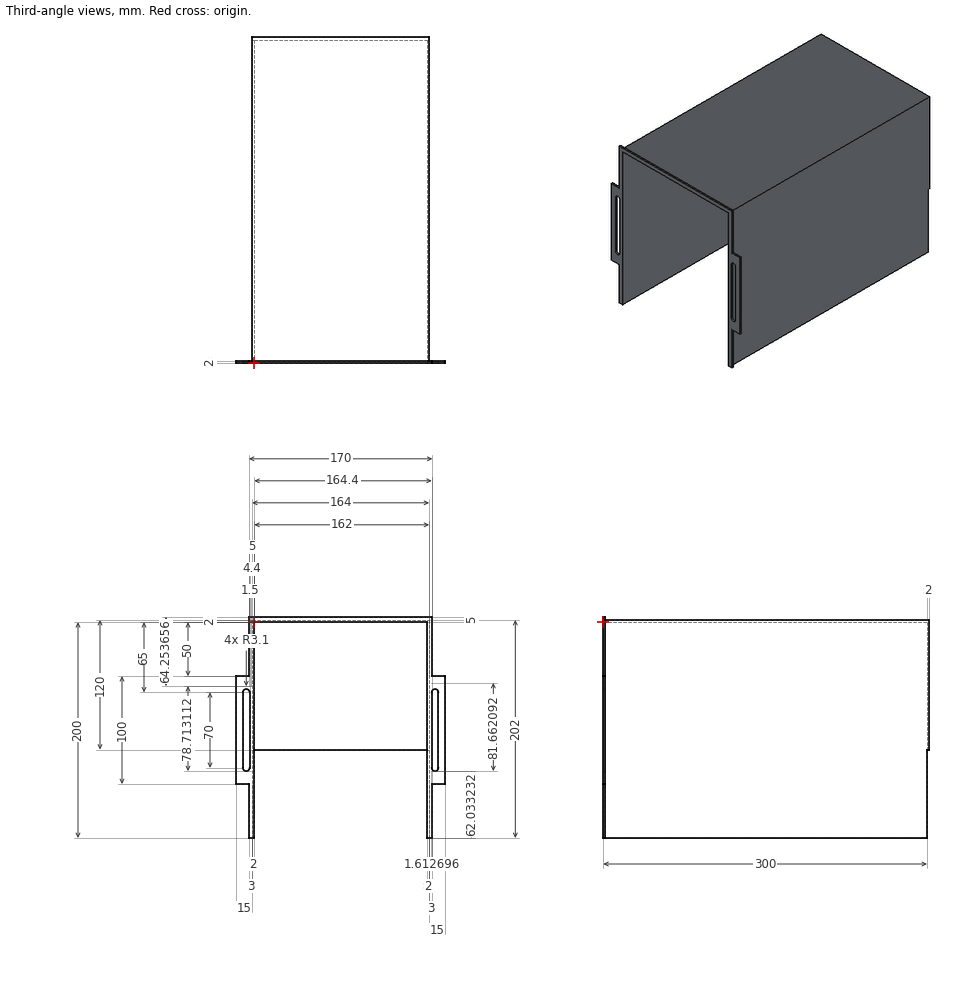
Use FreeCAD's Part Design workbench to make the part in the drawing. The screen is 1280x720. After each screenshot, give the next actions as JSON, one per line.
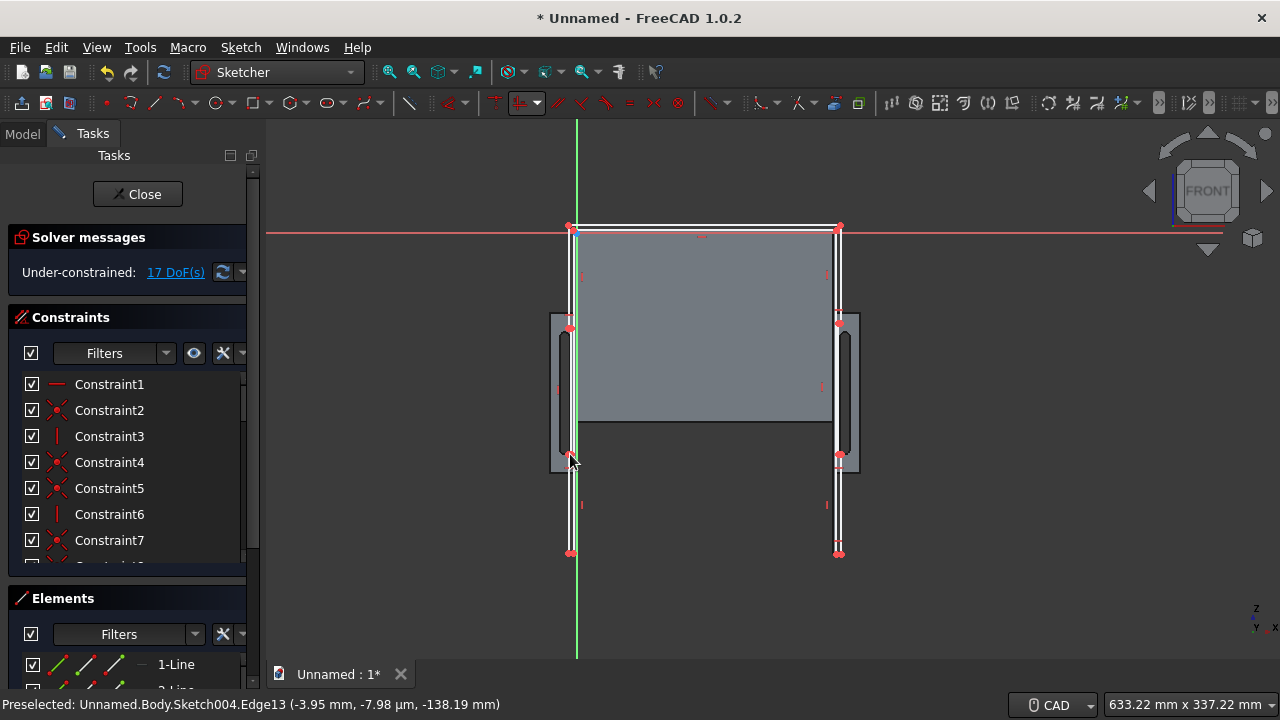
{"action": "scroll", "coordinate": [570, 554], "scroll_direction": "up", "scroll_amount": 12}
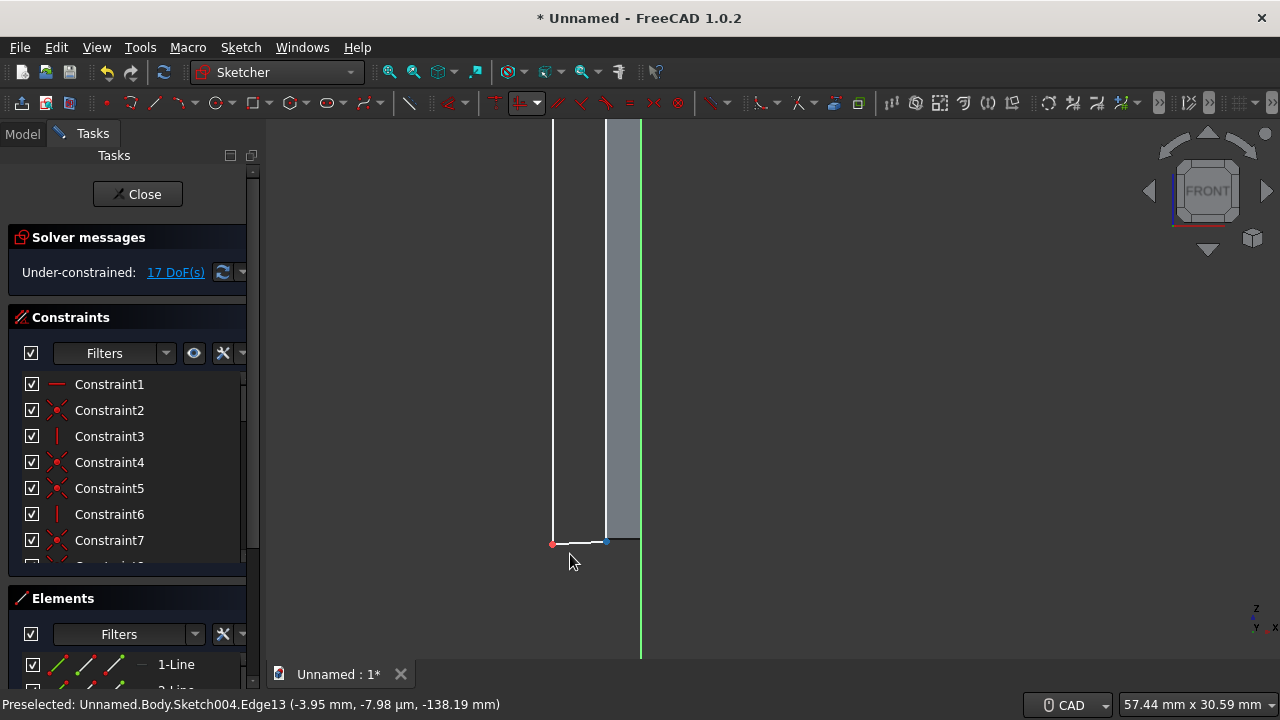
{"action": "left_click", "coordinate": [569, 544]}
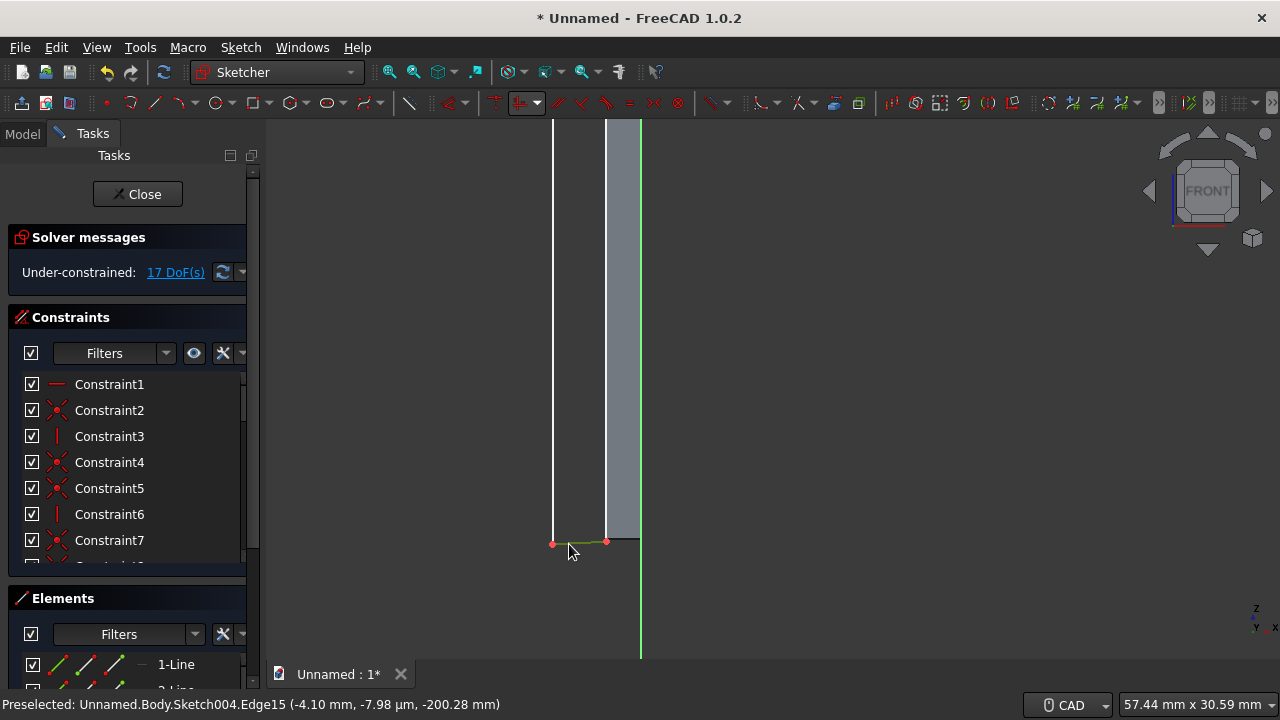
{"action": "left_click", "coordinate": [540, 104]}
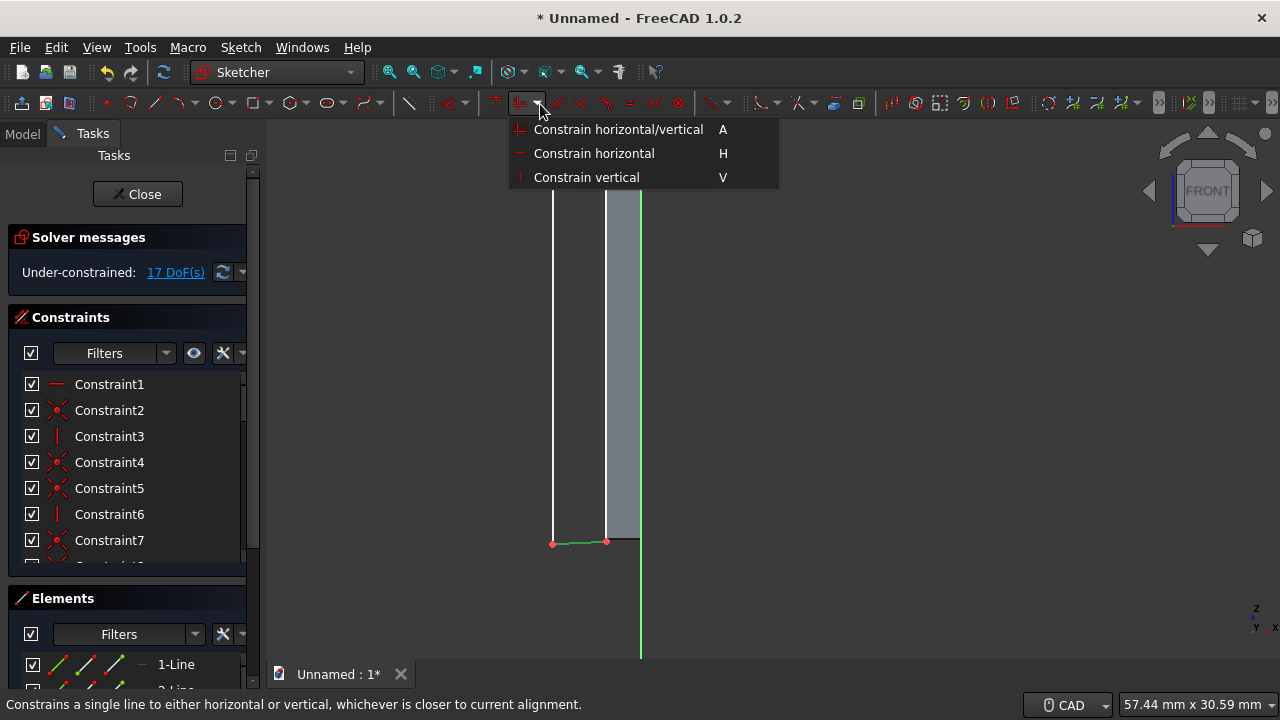
{"action": "left_click", "coordinate": [644, 153]}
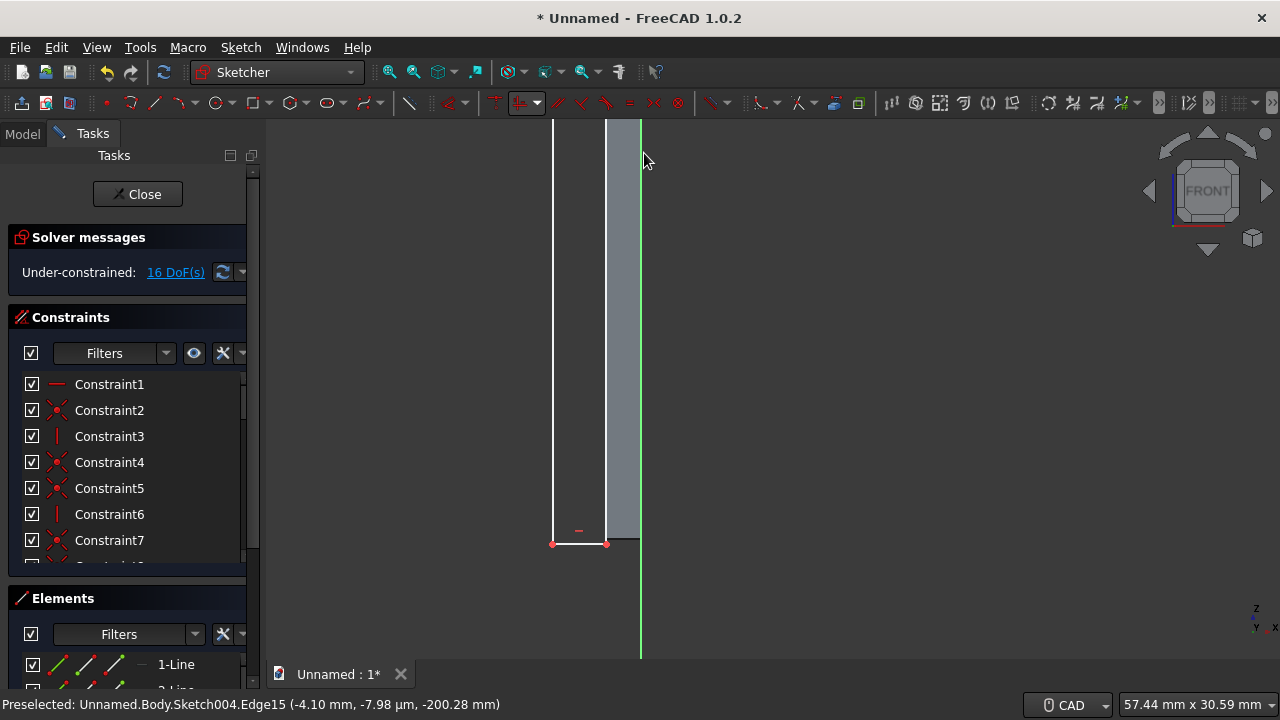
{"action": "left_click", "coordinate": [448, 104]}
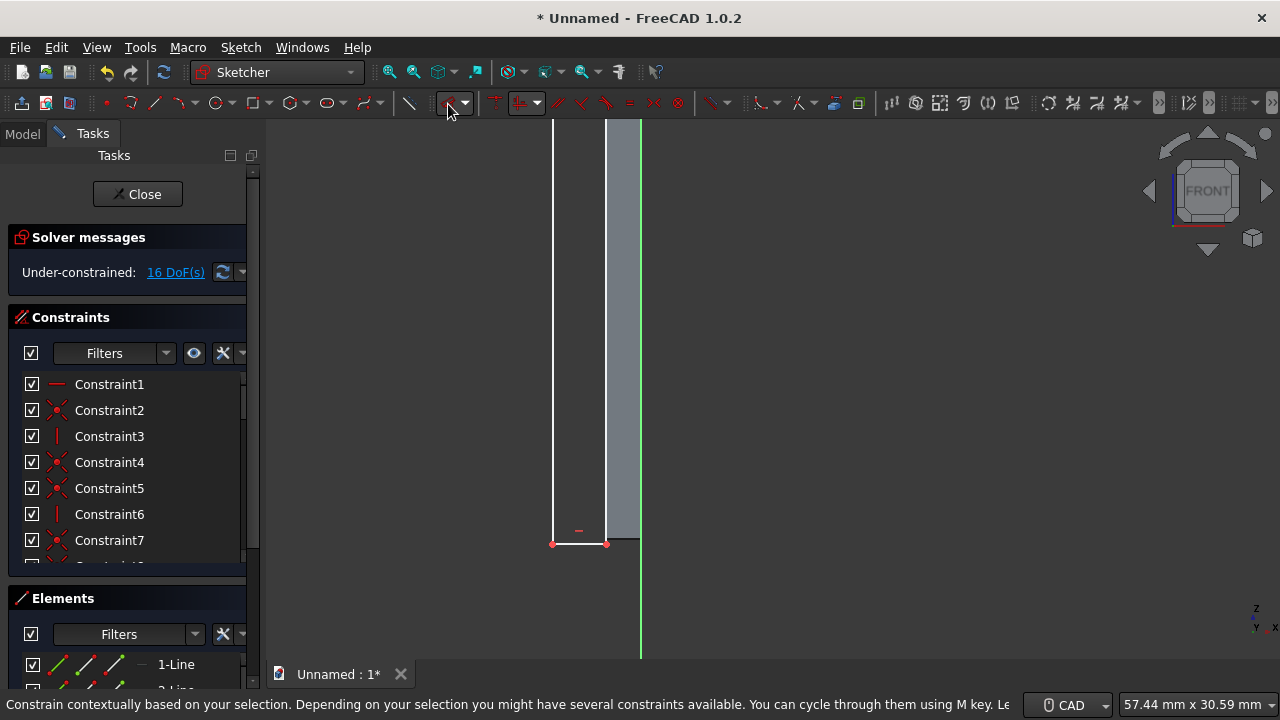
{"action": "scroll", "coordinate": [570, 555], "scroll_direction": "down", "scroll_amount": 12}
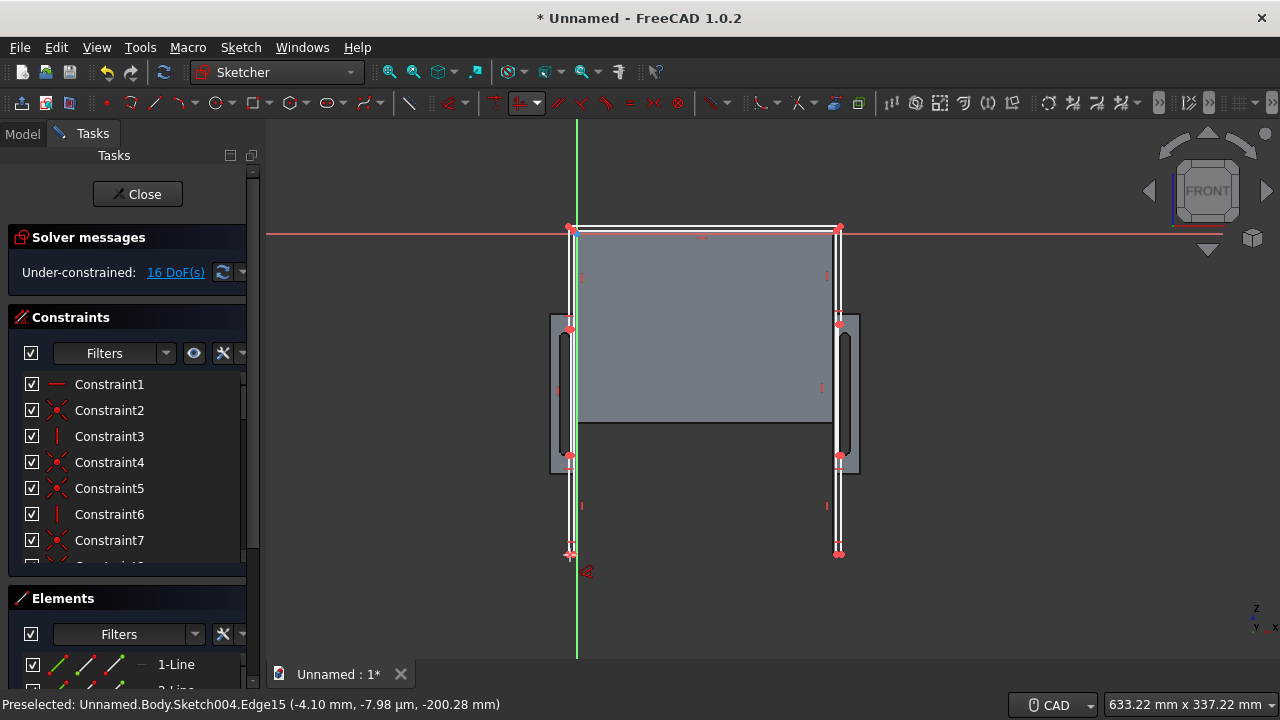
{"action": "scroll", "coordinate": [838, 555], "scroll_direction": "up", "scroll_amount": 12}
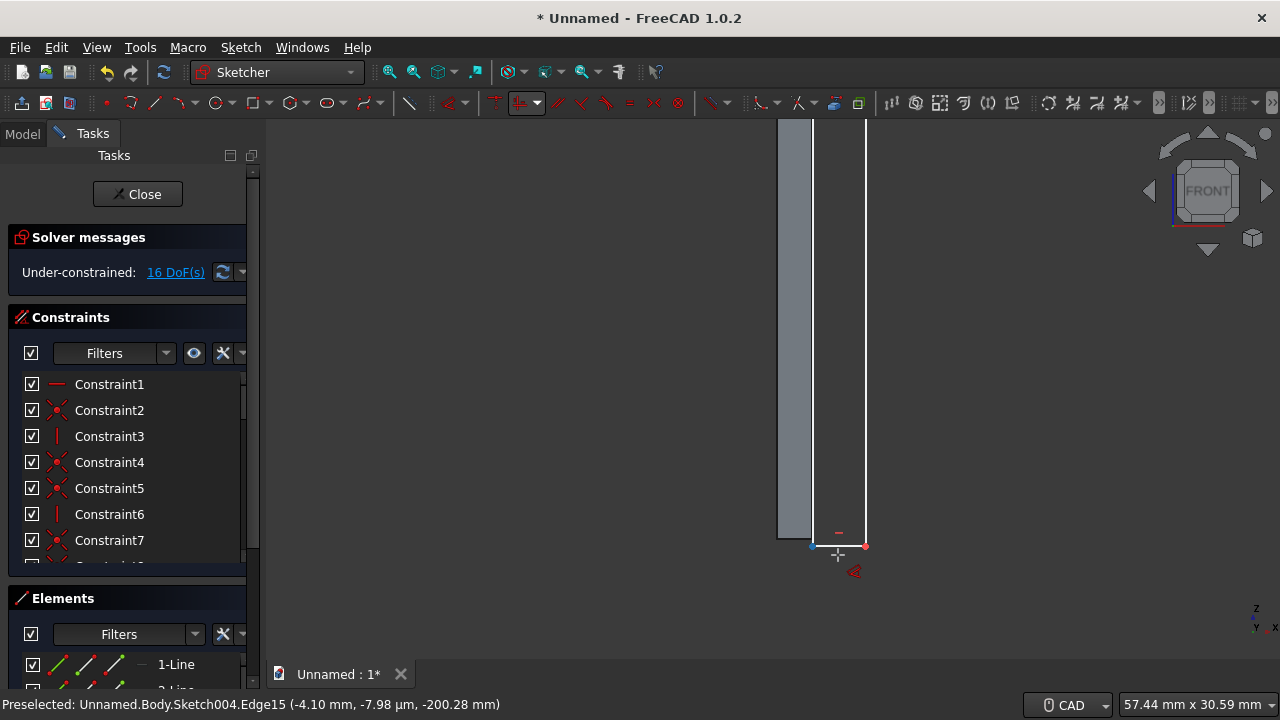
{"action": "left_click", "coordinate": [829, 546]}
{"action": "left_click", "coordinate": [839, 580]}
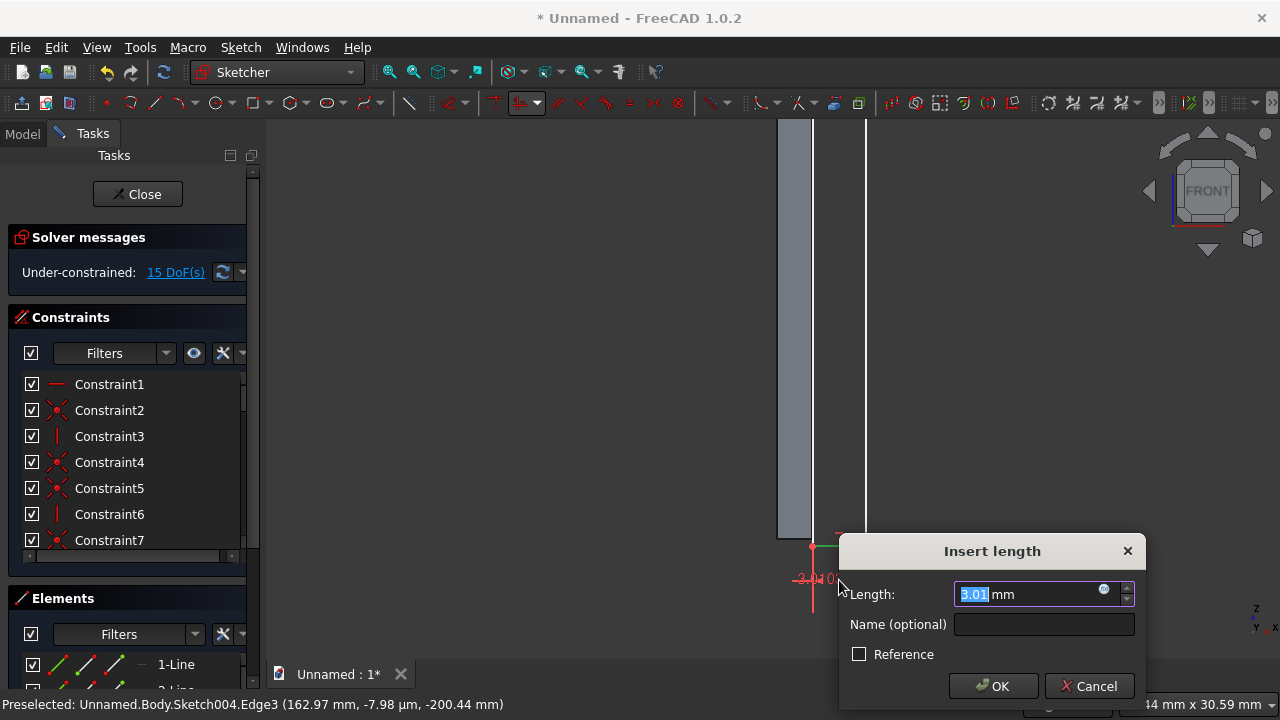
{"action": "type", "text": "3"}
{"action": "key", "text": "Return"}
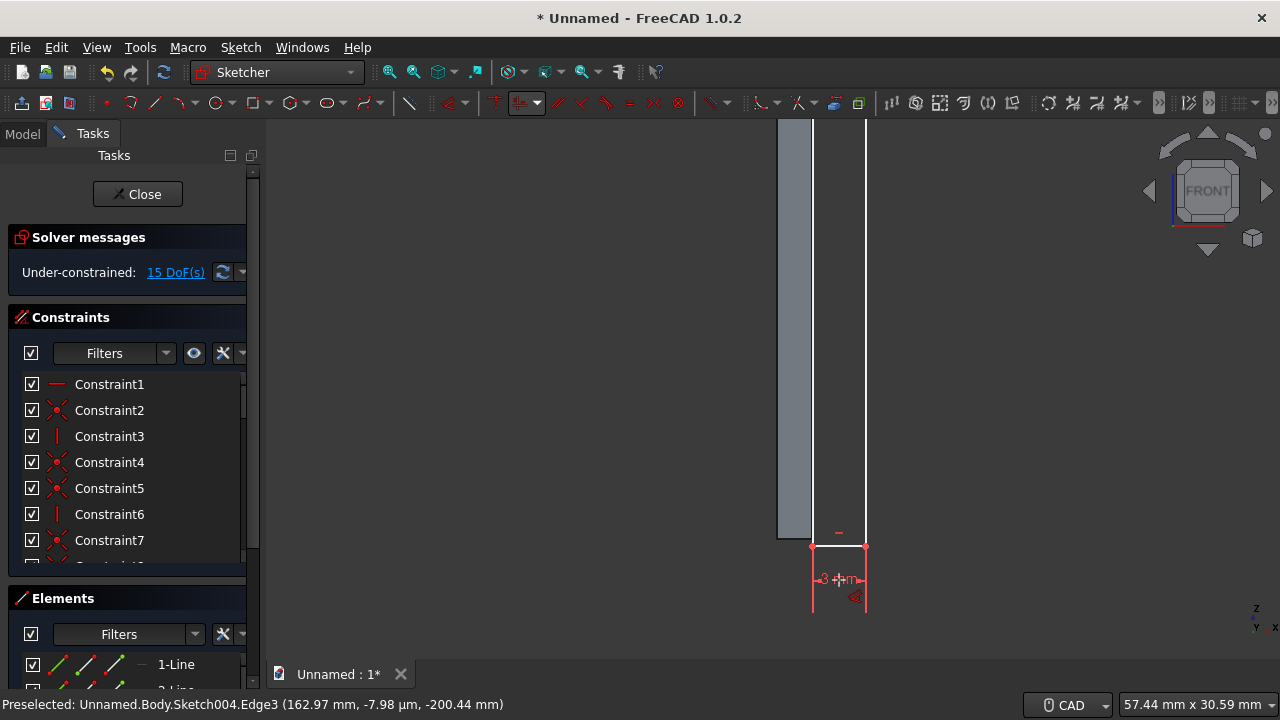
{"action": "scroll", "coordinate": [838, 555], "scroll_direction": "down", "scroll_amount": 12}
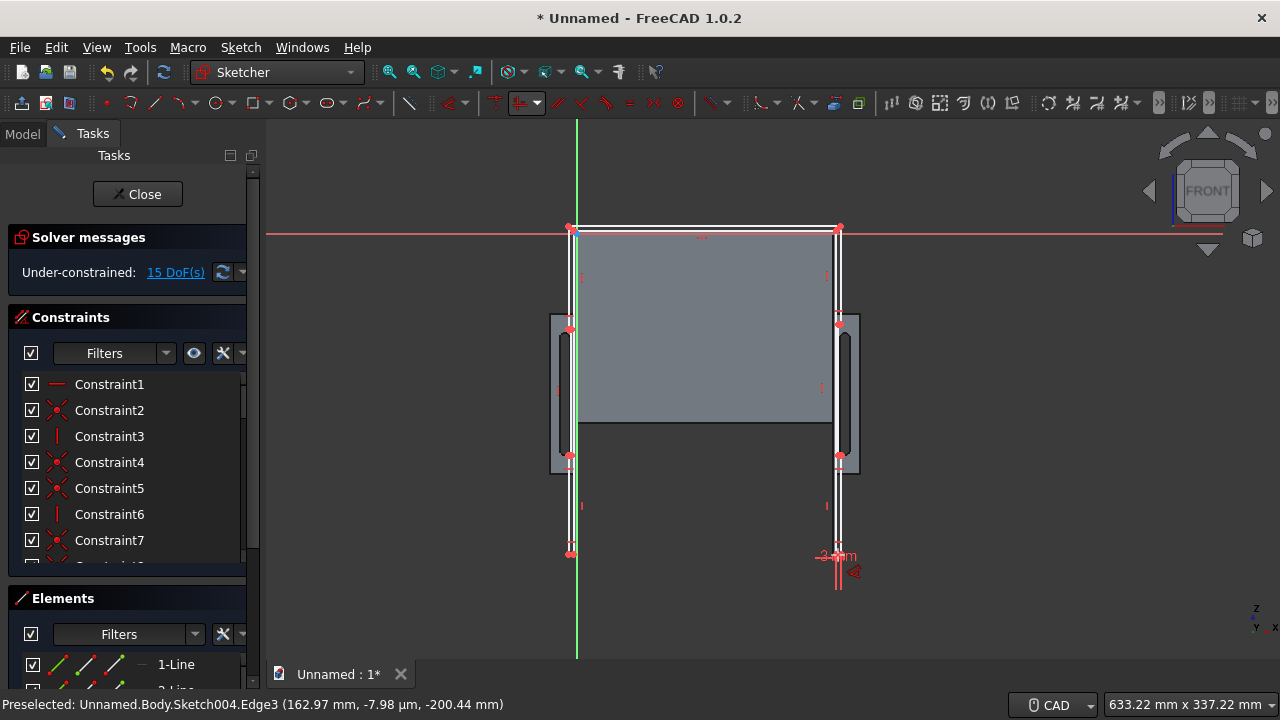
{"action": "scroll", "coordinate": [570, 555], "scroll_direction": "up", "scroll_amount": 12}